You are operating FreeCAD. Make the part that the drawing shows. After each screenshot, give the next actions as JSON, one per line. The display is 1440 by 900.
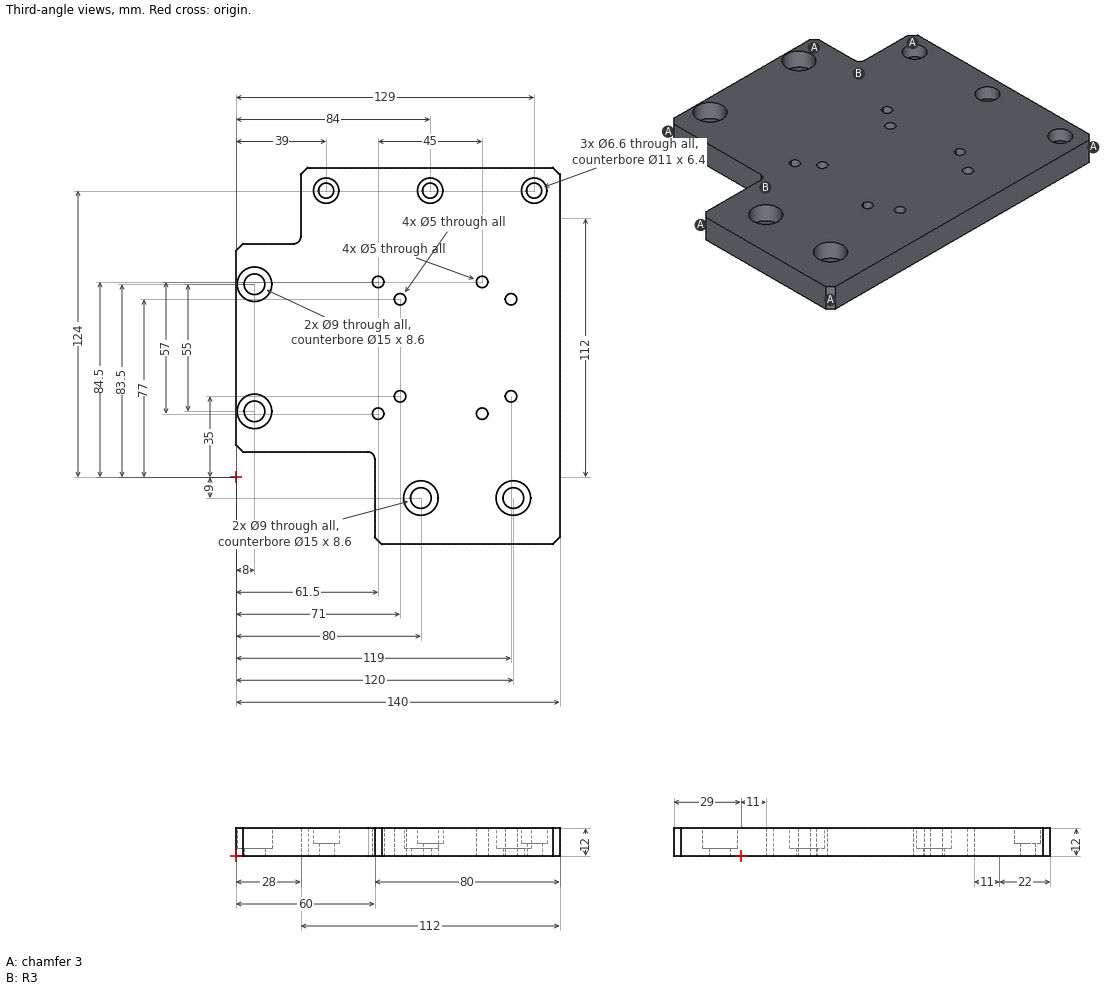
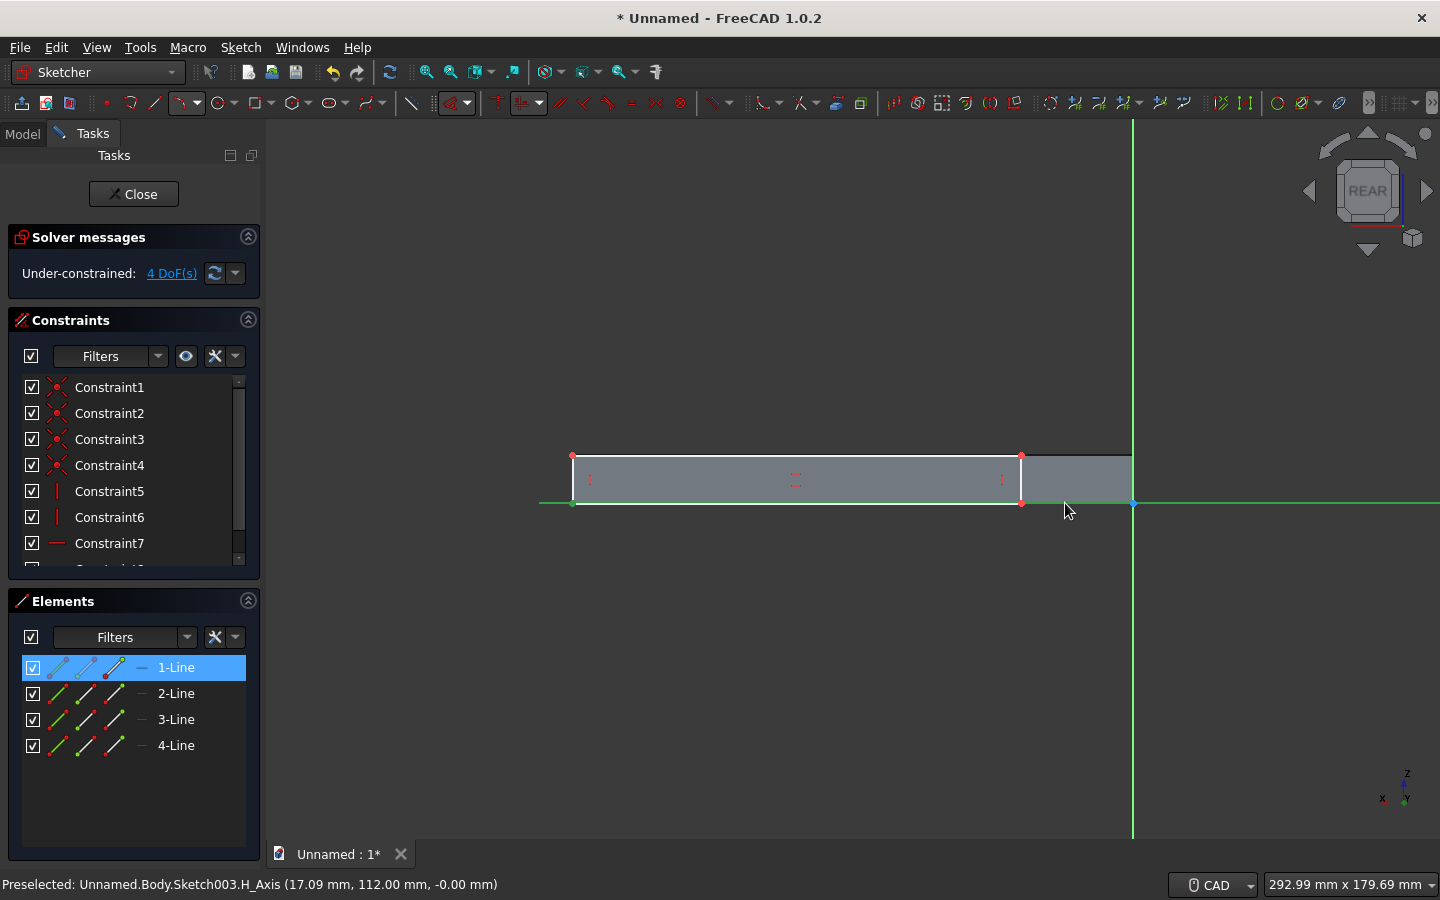
{"action": "left_click", "coordinate": [498, 104]}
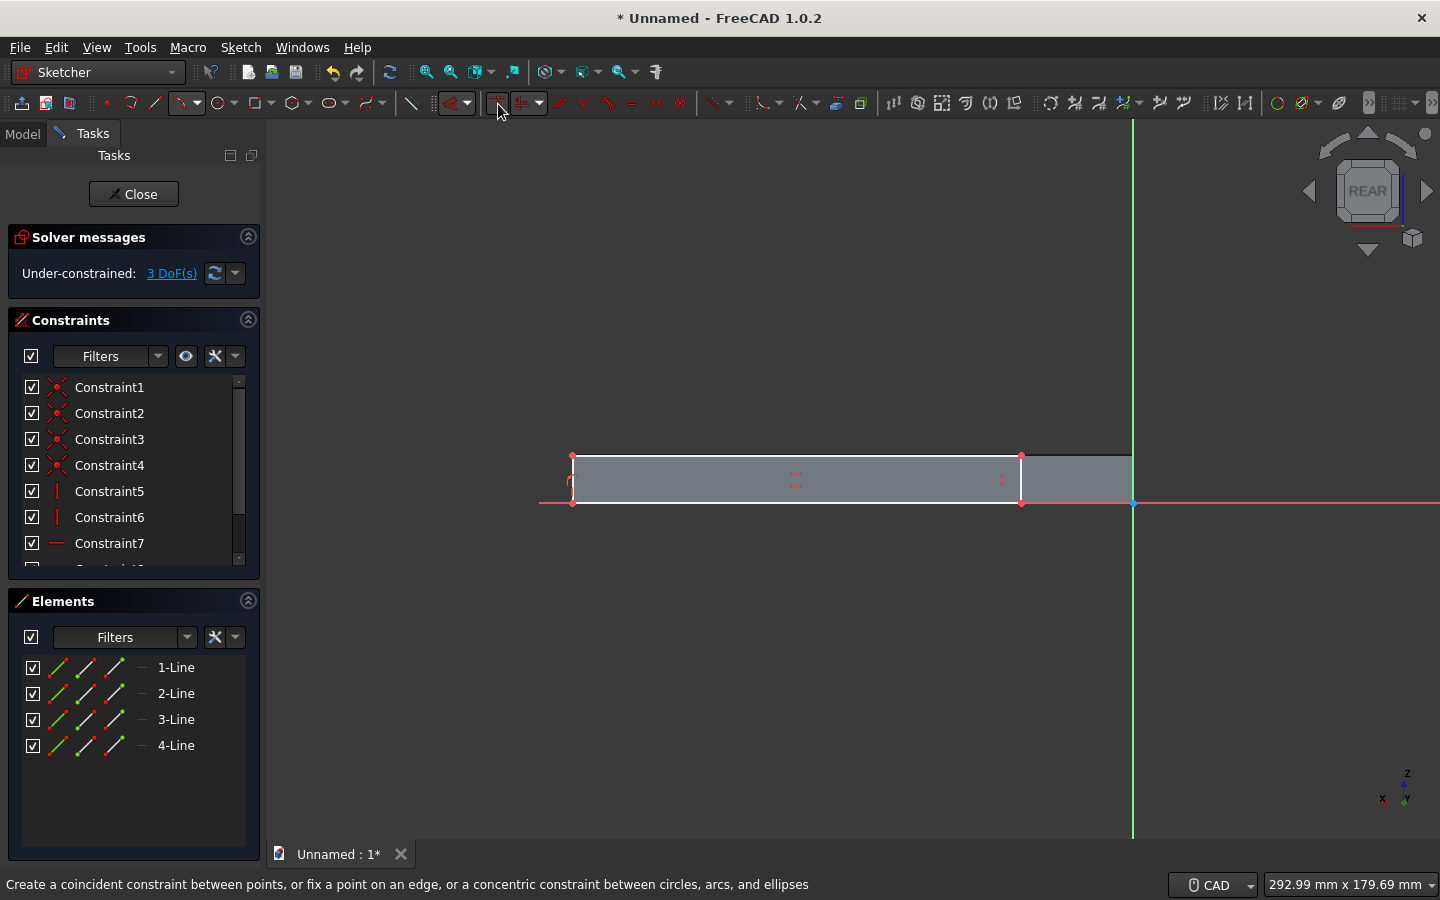
{"action": "left_click", "coordinate": [573, 470]}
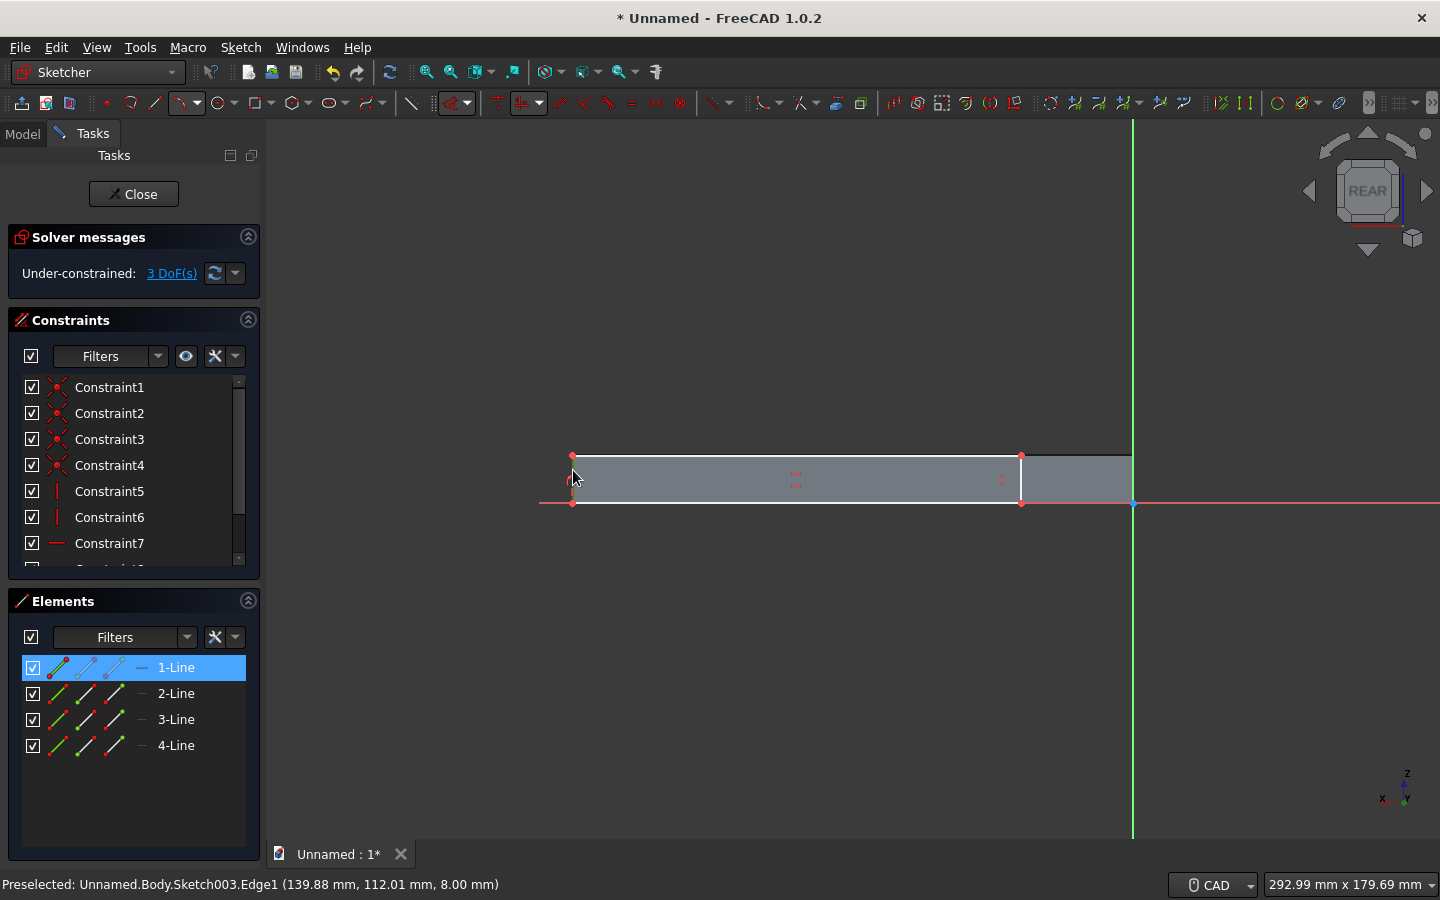
{"action": "key", "text": "i"}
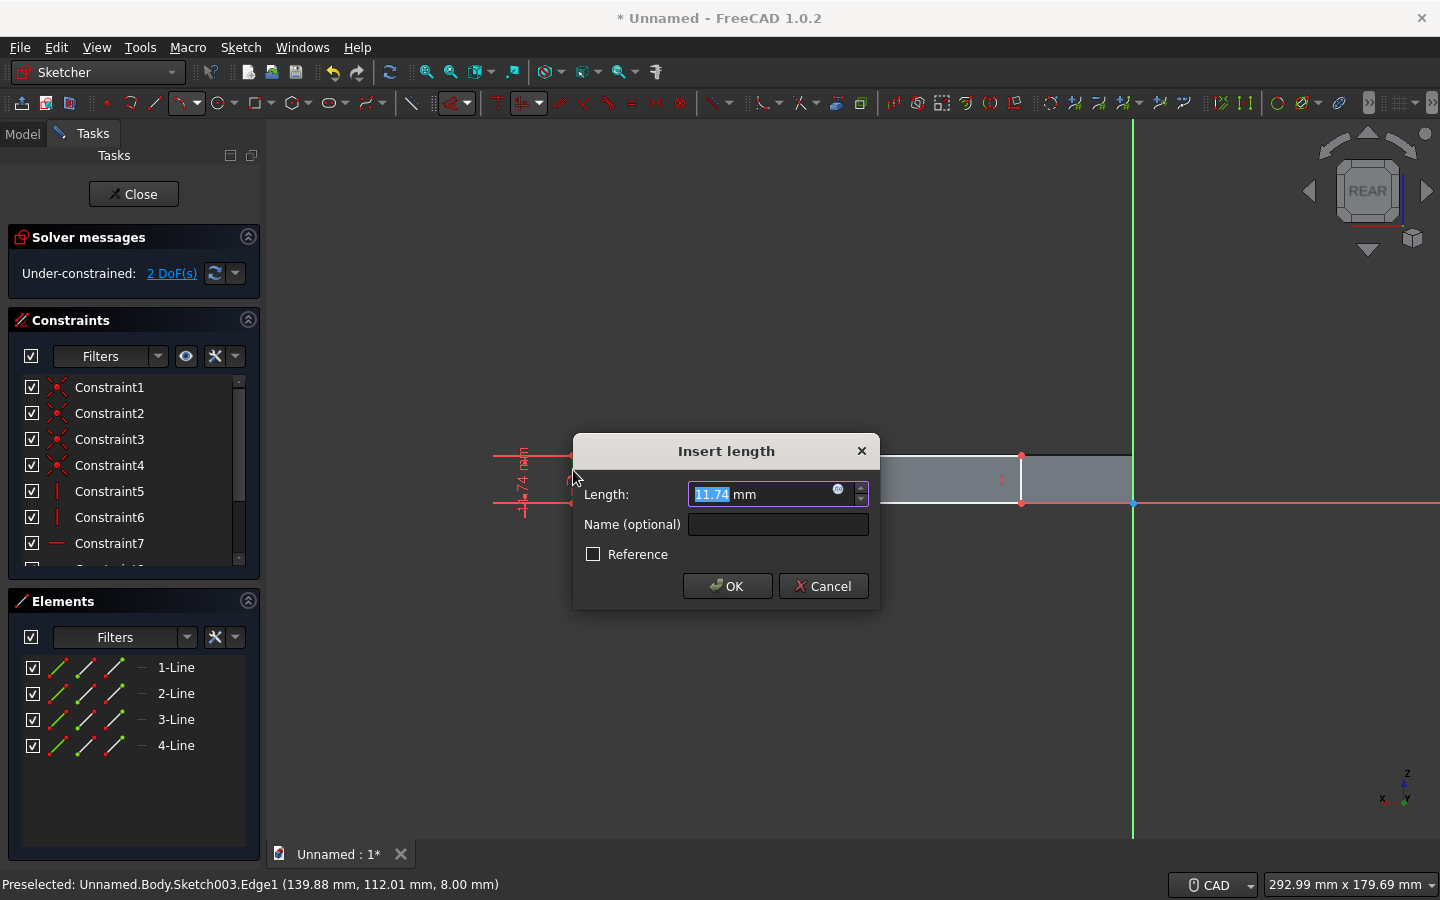
{"action": "type", "text": "12"}
{"action": "key", "text": "Return"}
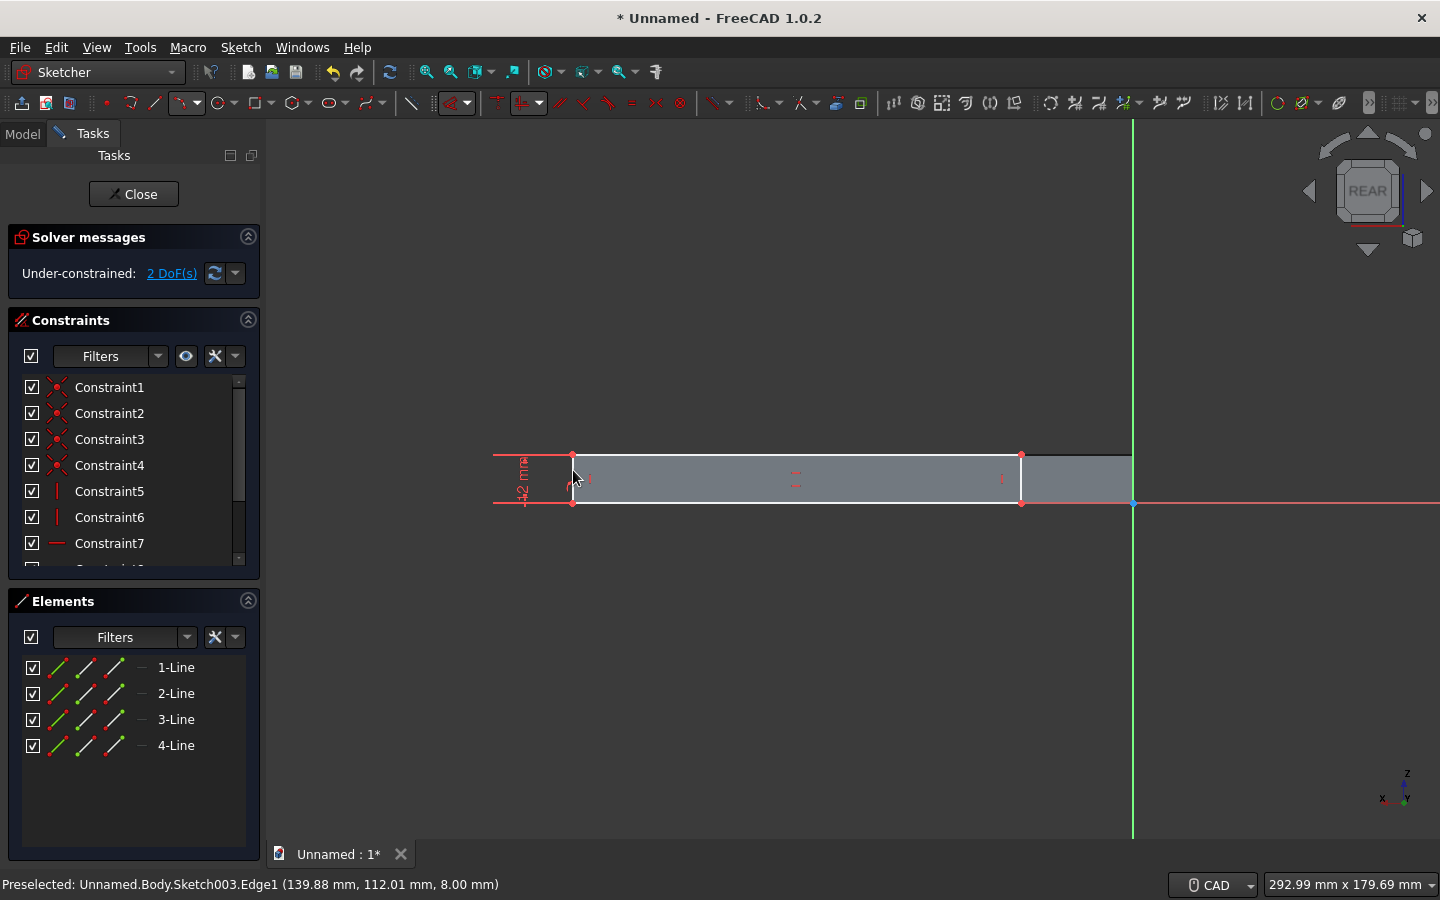
{"action": "left_click", "coordinate": [707, 503]}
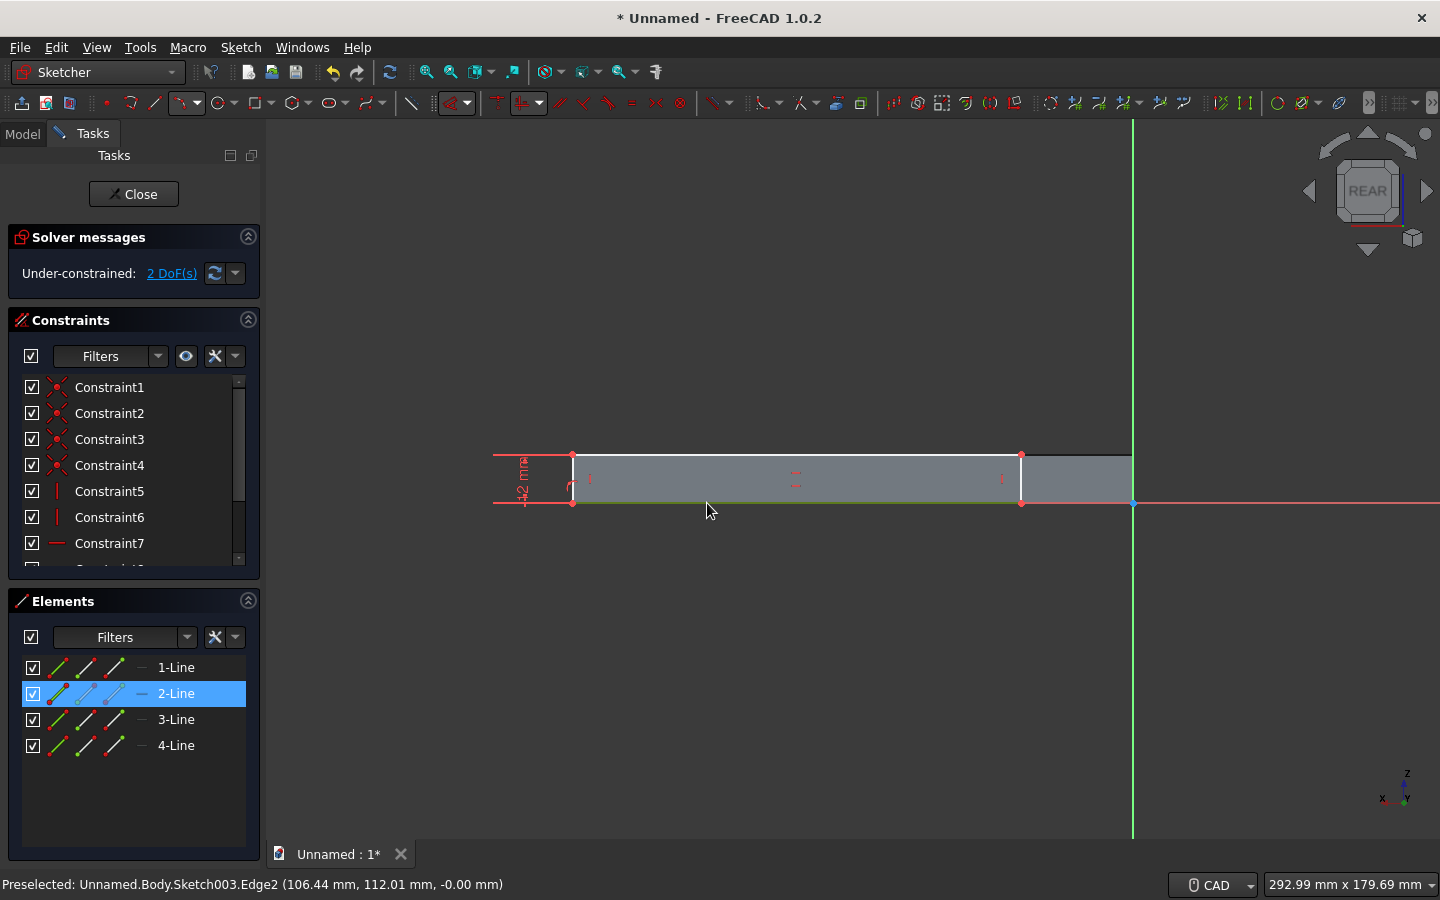
{"action": "left_click", "coordinate": [470, 104]}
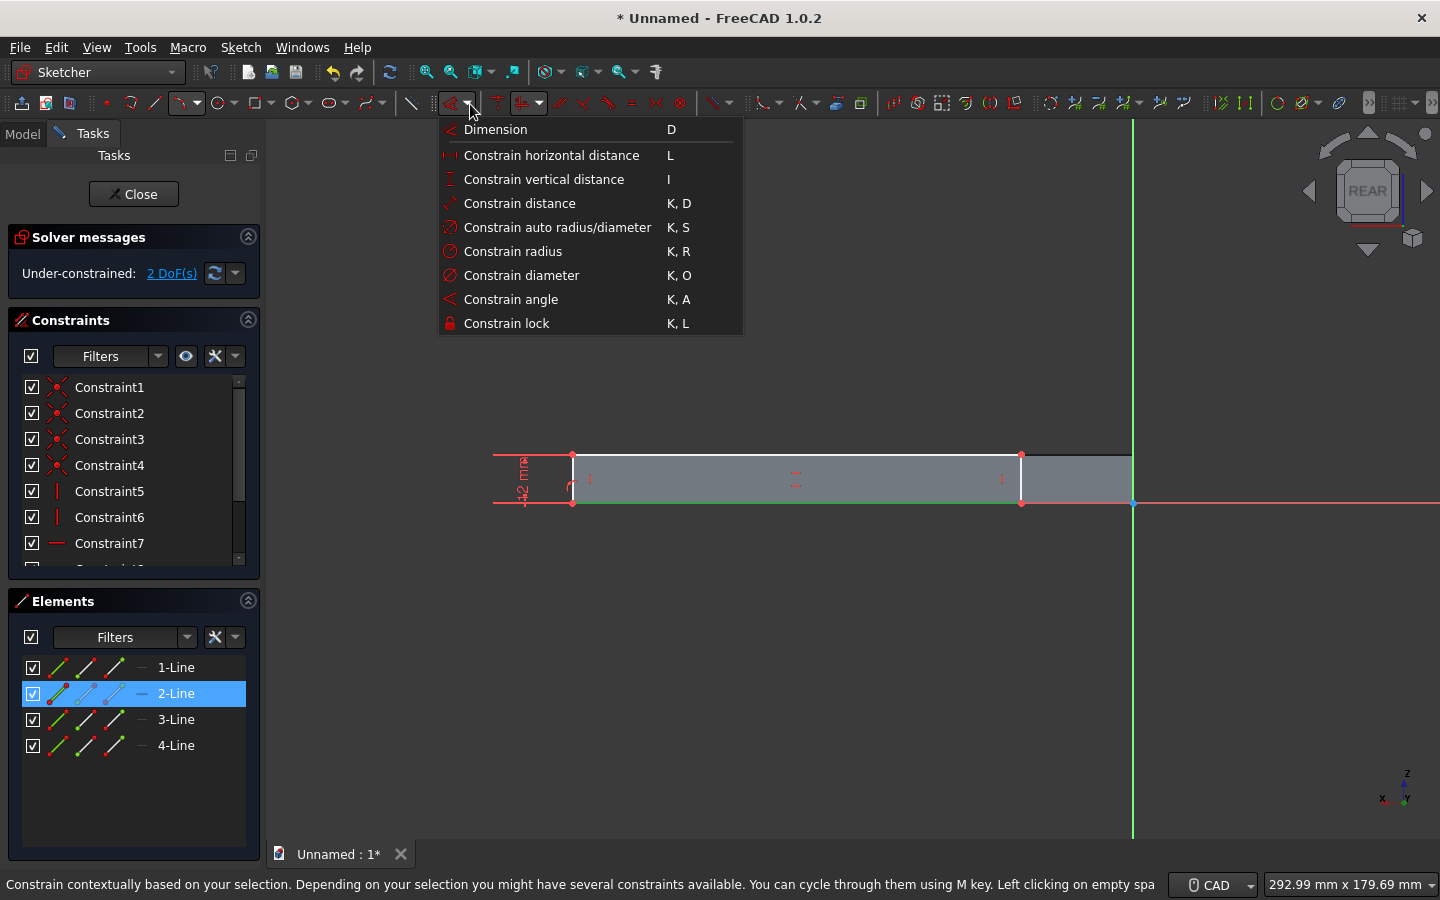
{"action": "left_click", "coordinate": [591, 155]}